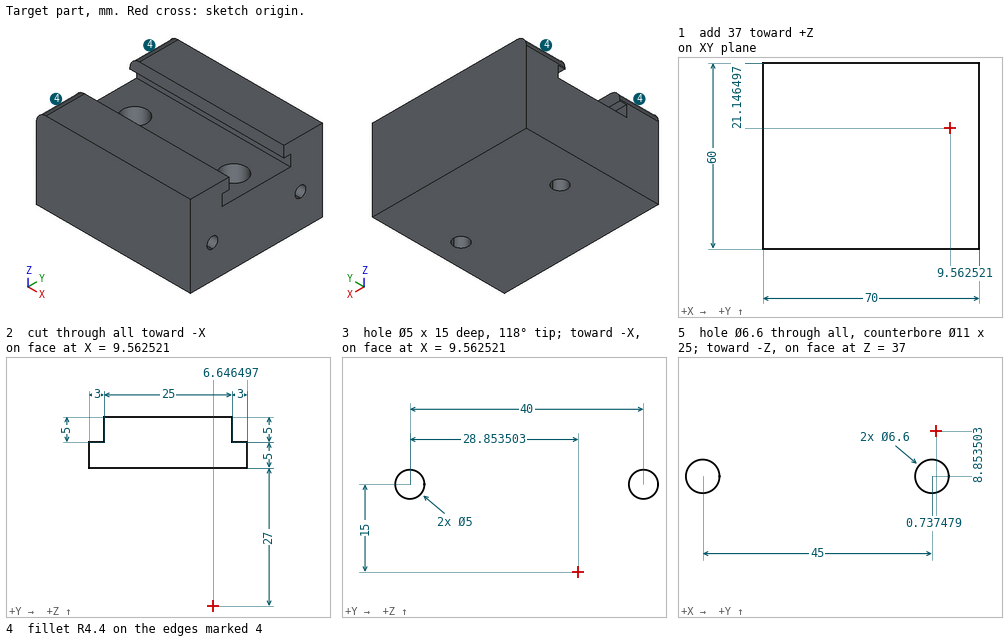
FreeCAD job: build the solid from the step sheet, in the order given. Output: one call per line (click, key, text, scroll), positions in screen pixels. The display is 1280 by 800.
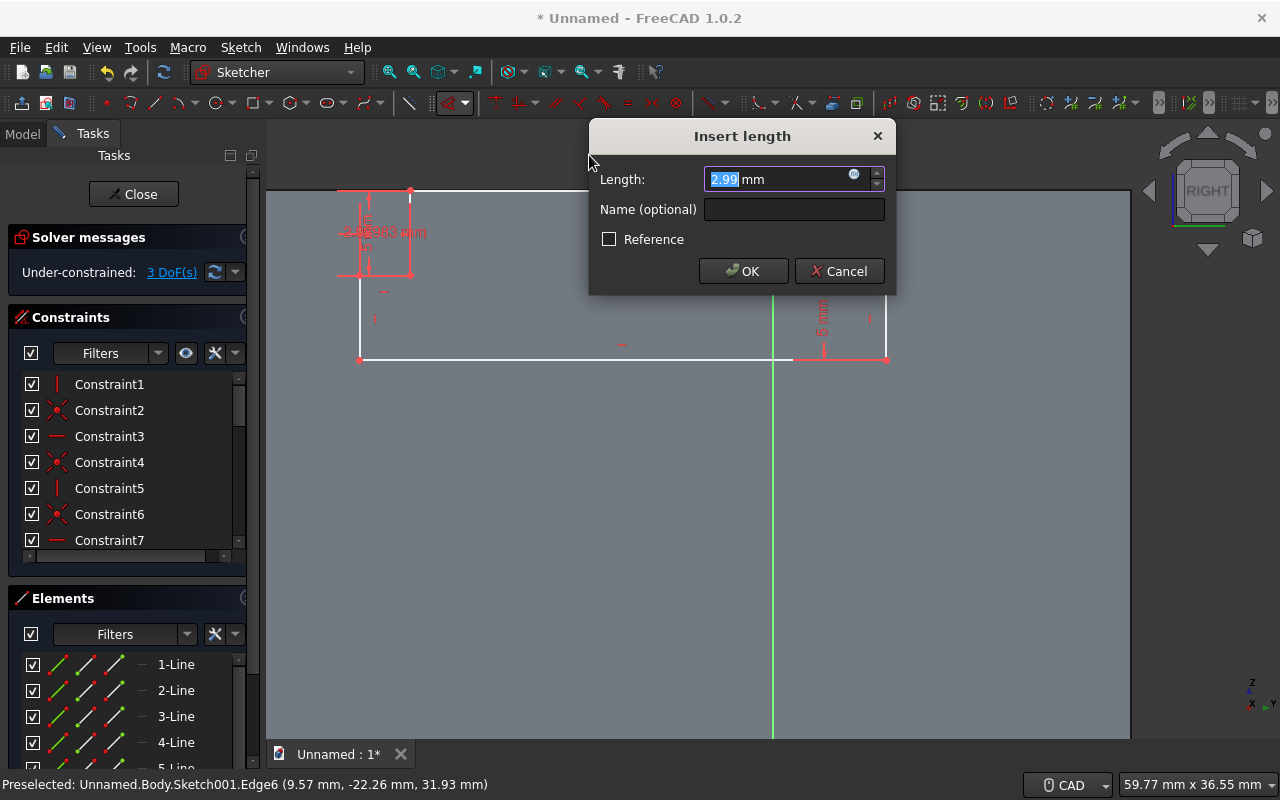
text(3)
key(Return)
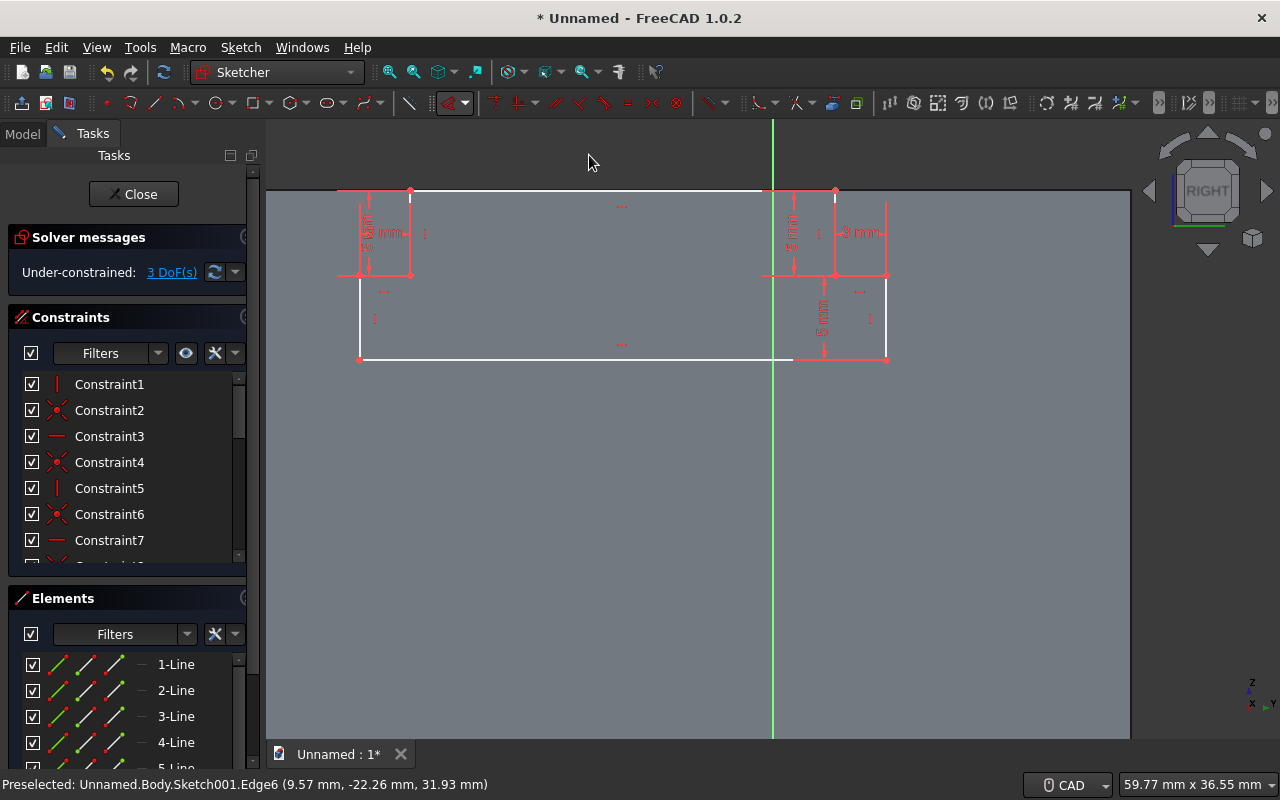
click(708, 191)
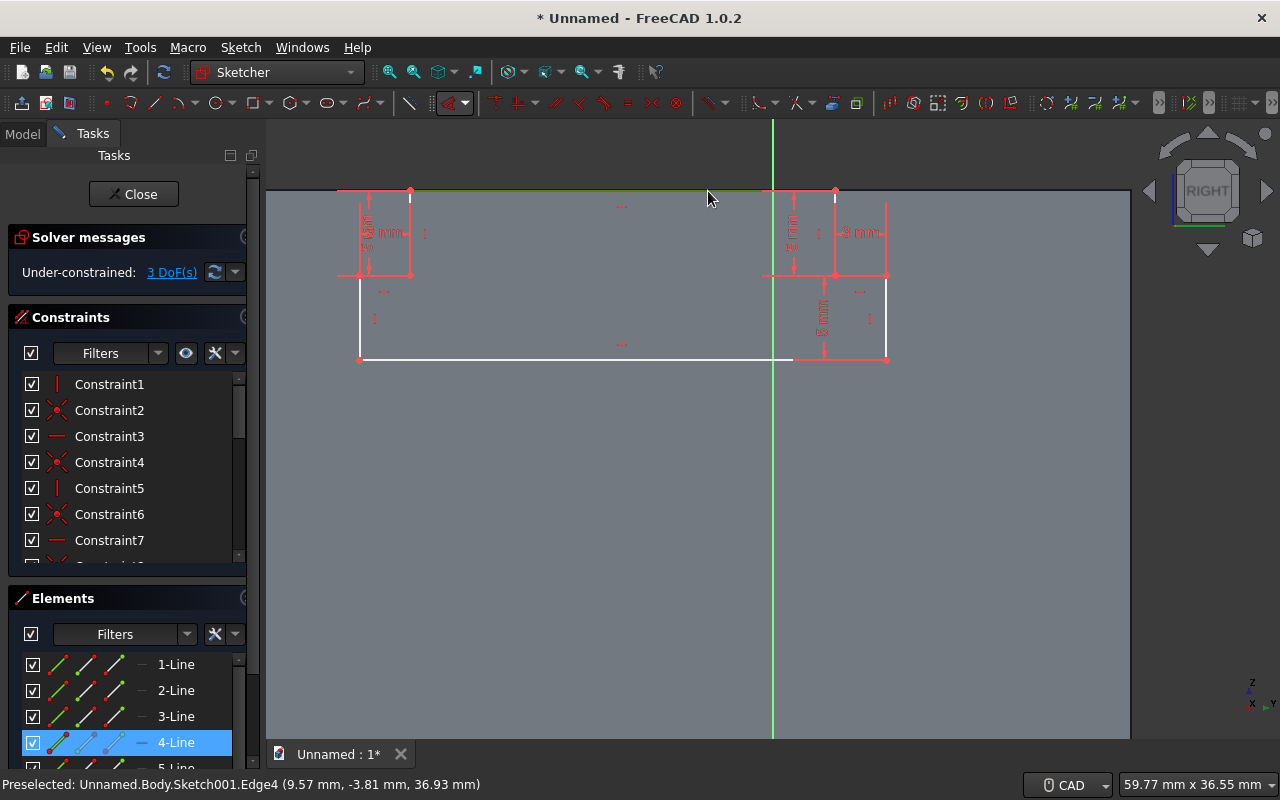
key(l)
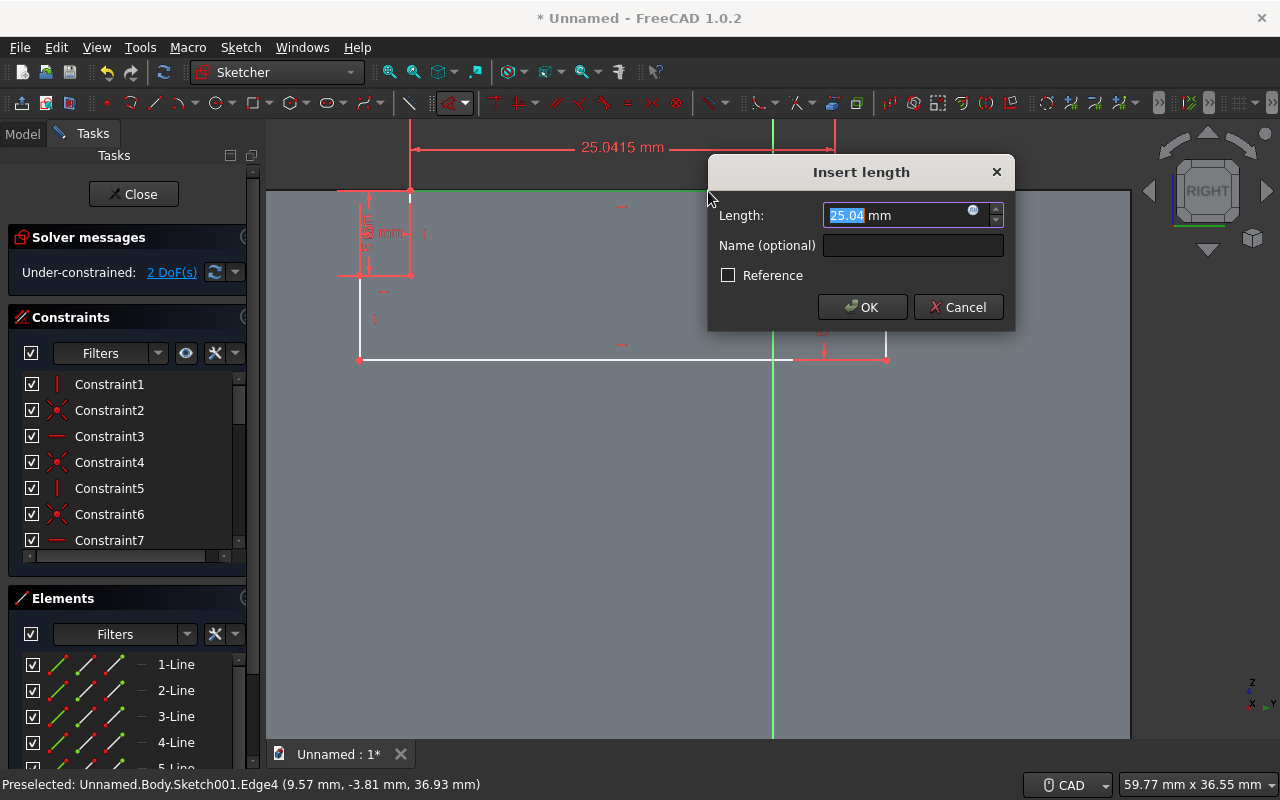
text(25)
key(Return)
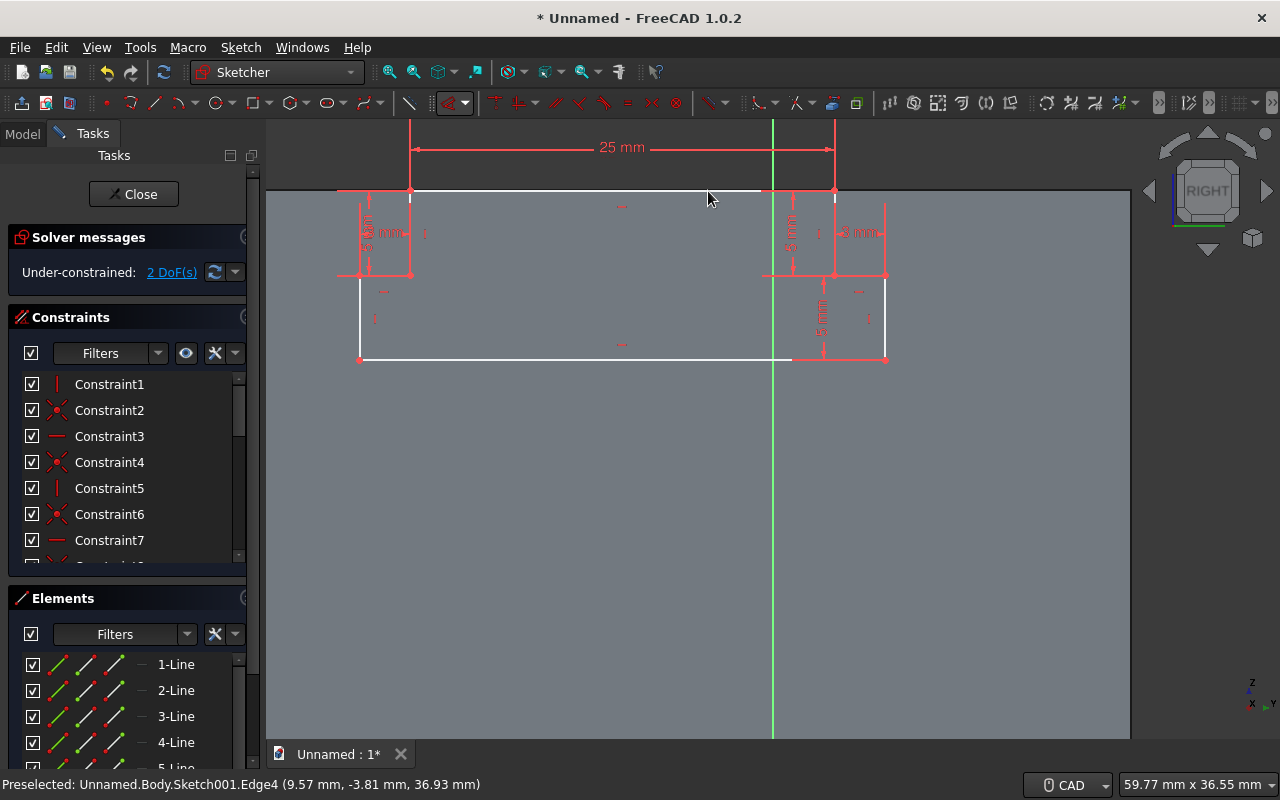
click(885, 360)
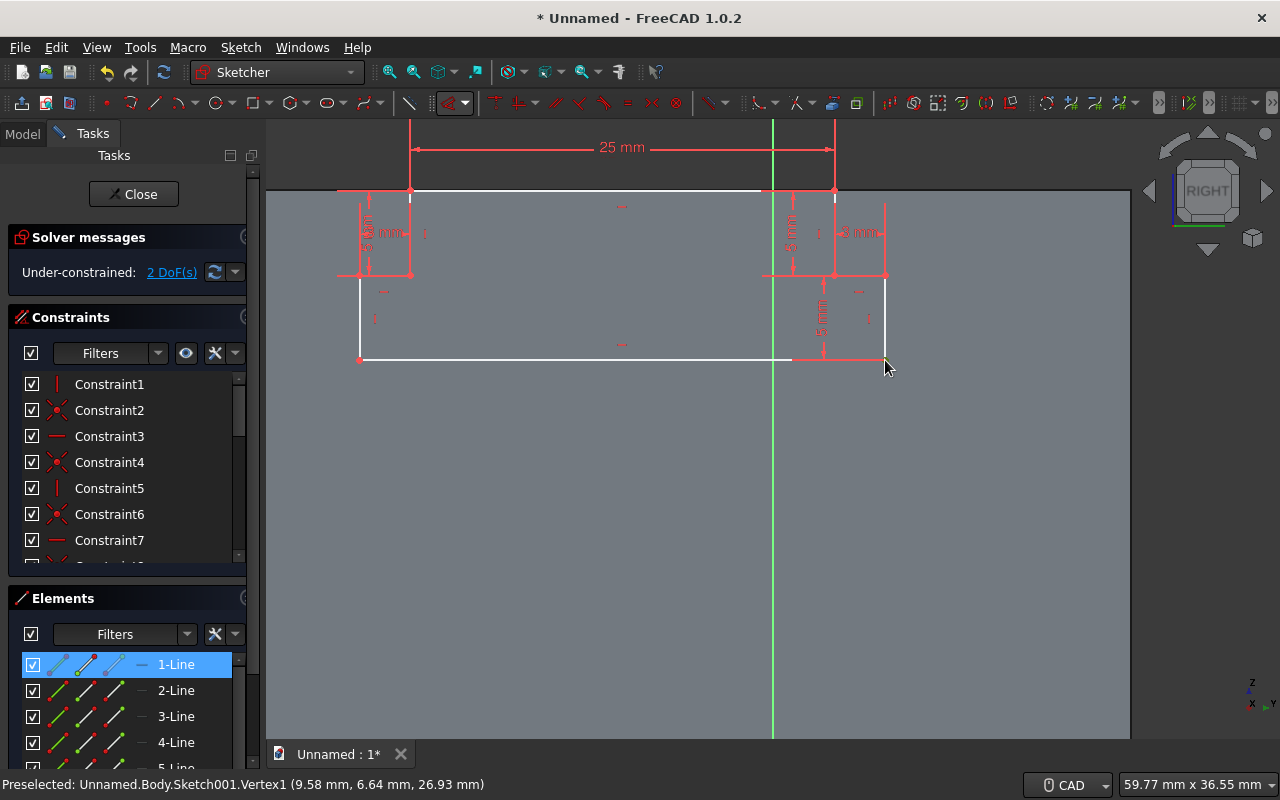
key(i)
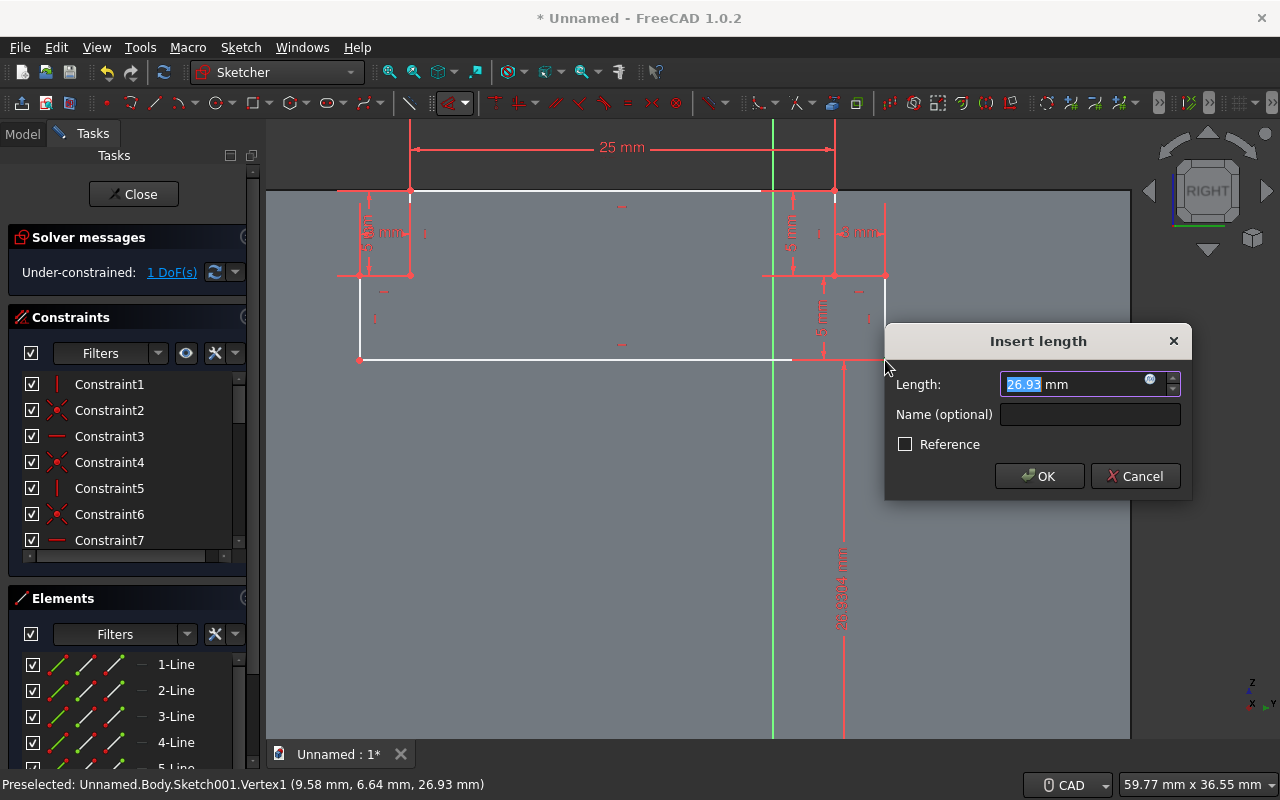
text(27)
key(Return)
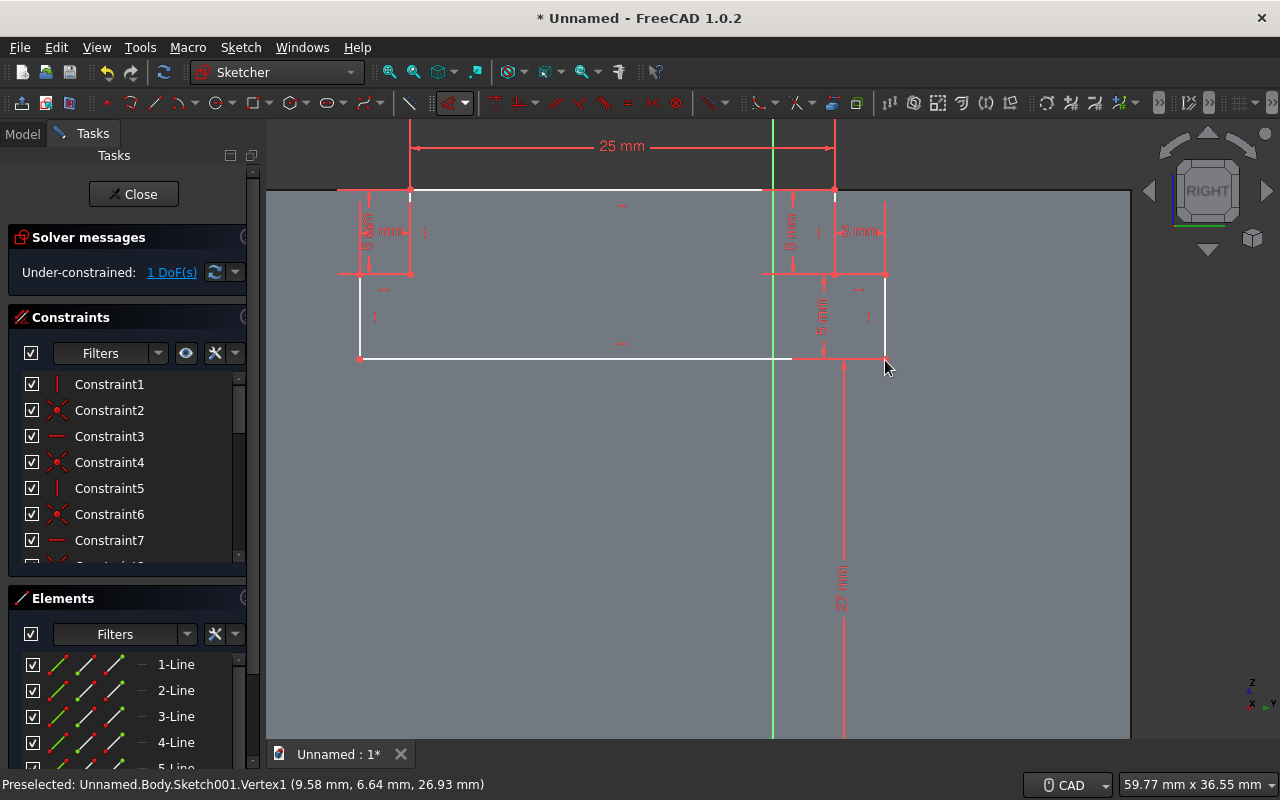
click(885, 359)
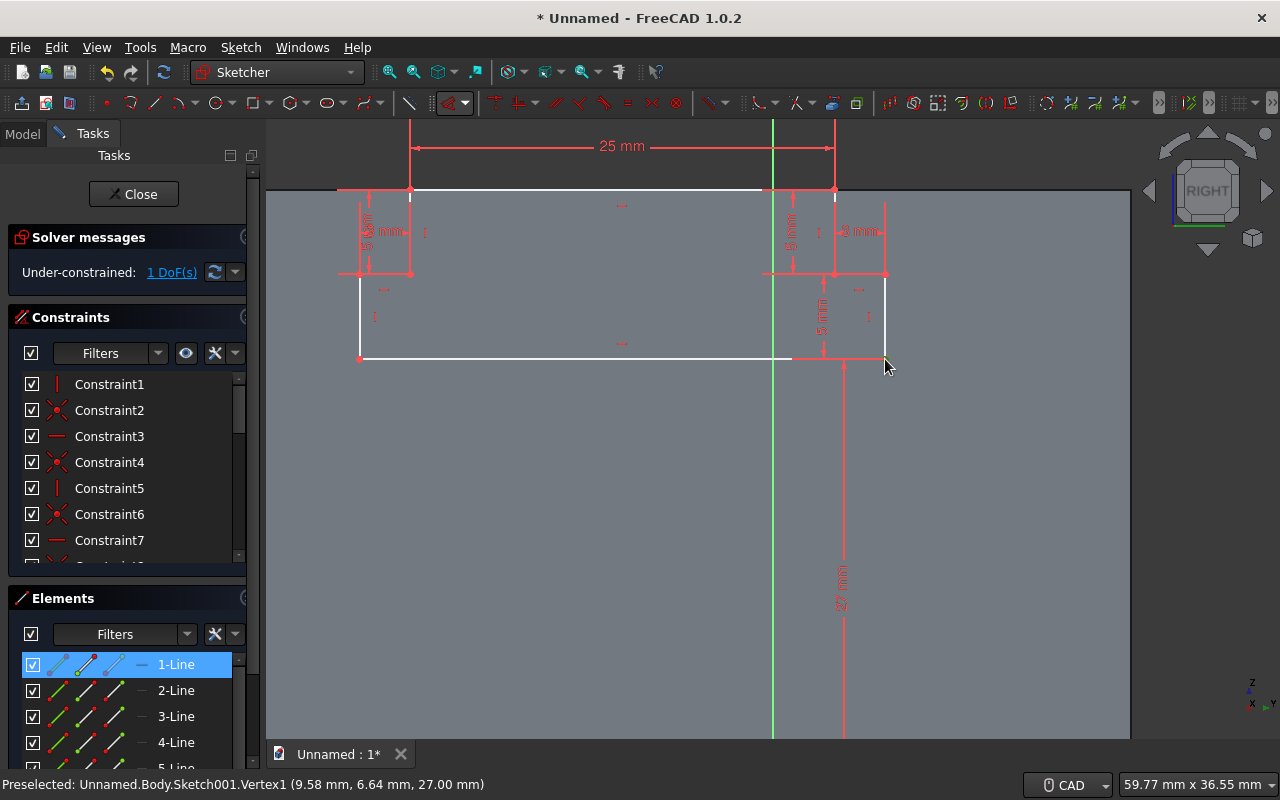
click(468, 104)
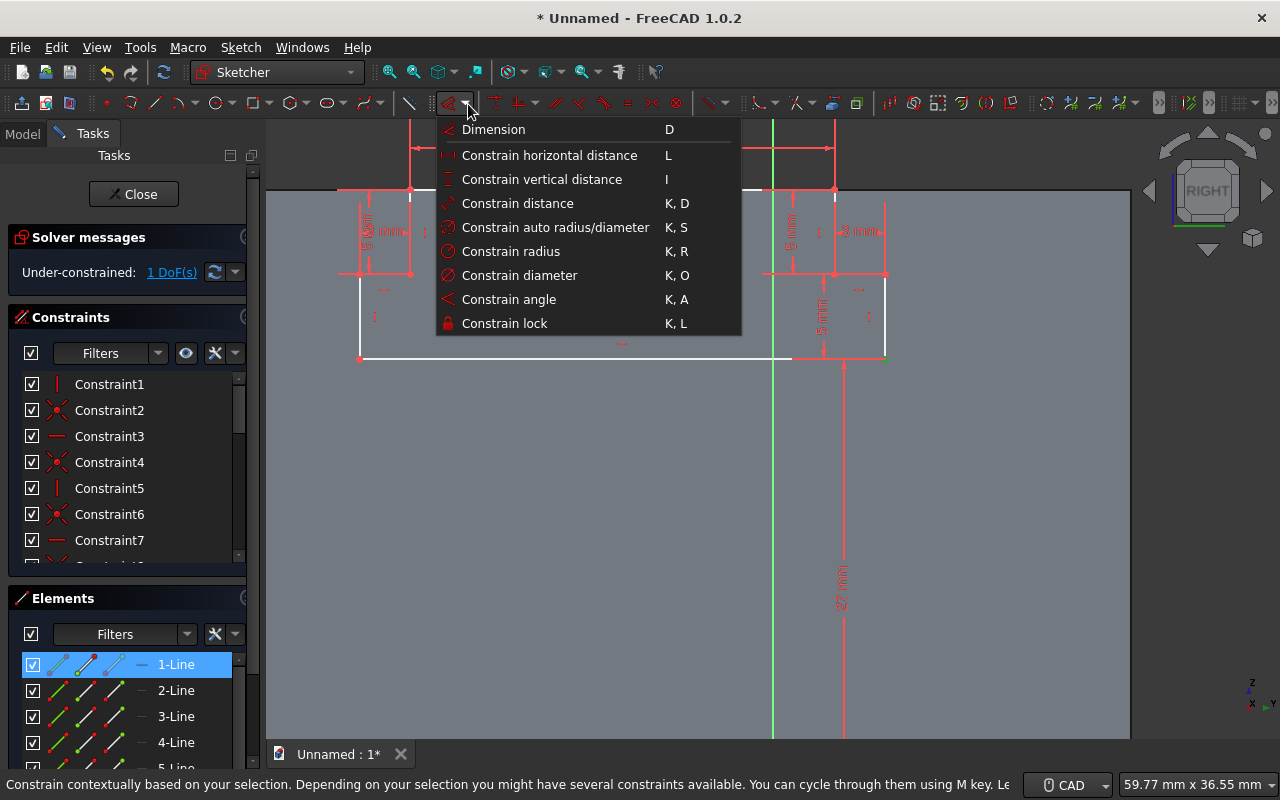
click(589, 155)